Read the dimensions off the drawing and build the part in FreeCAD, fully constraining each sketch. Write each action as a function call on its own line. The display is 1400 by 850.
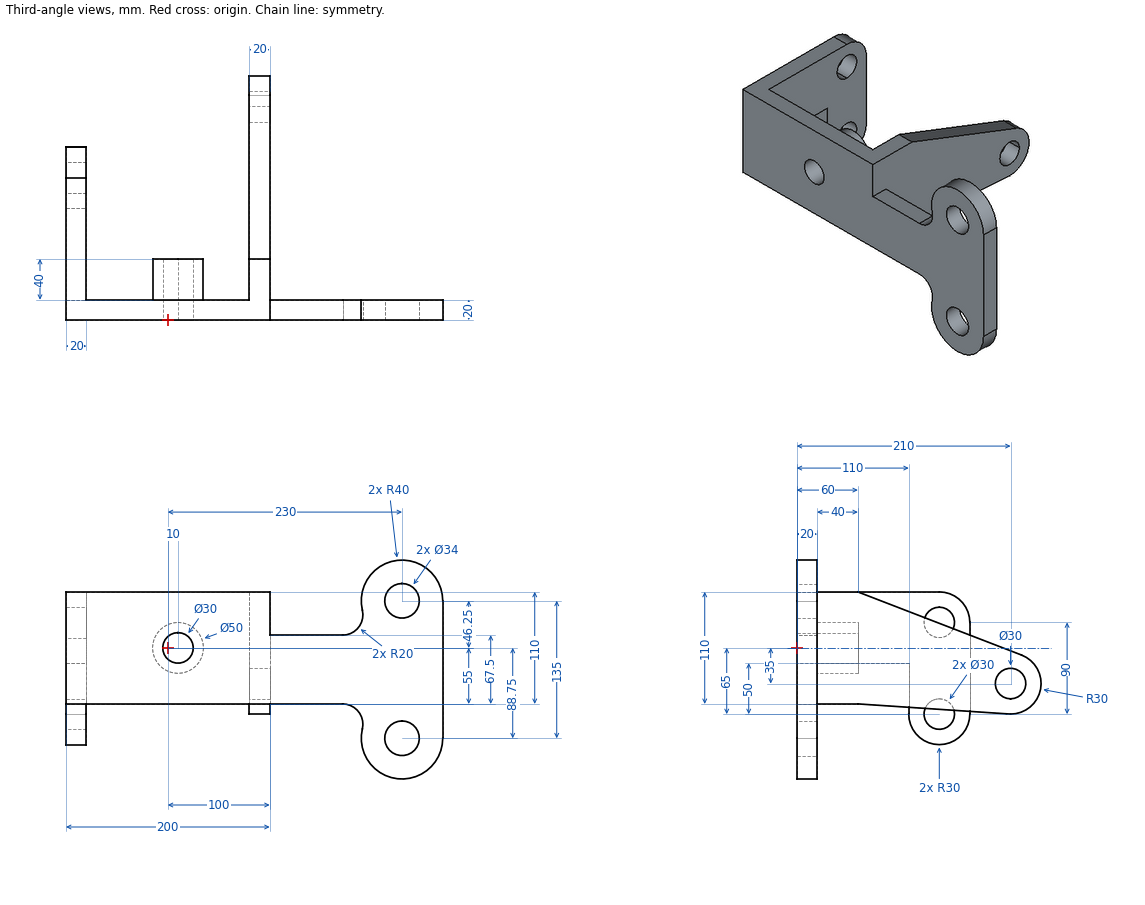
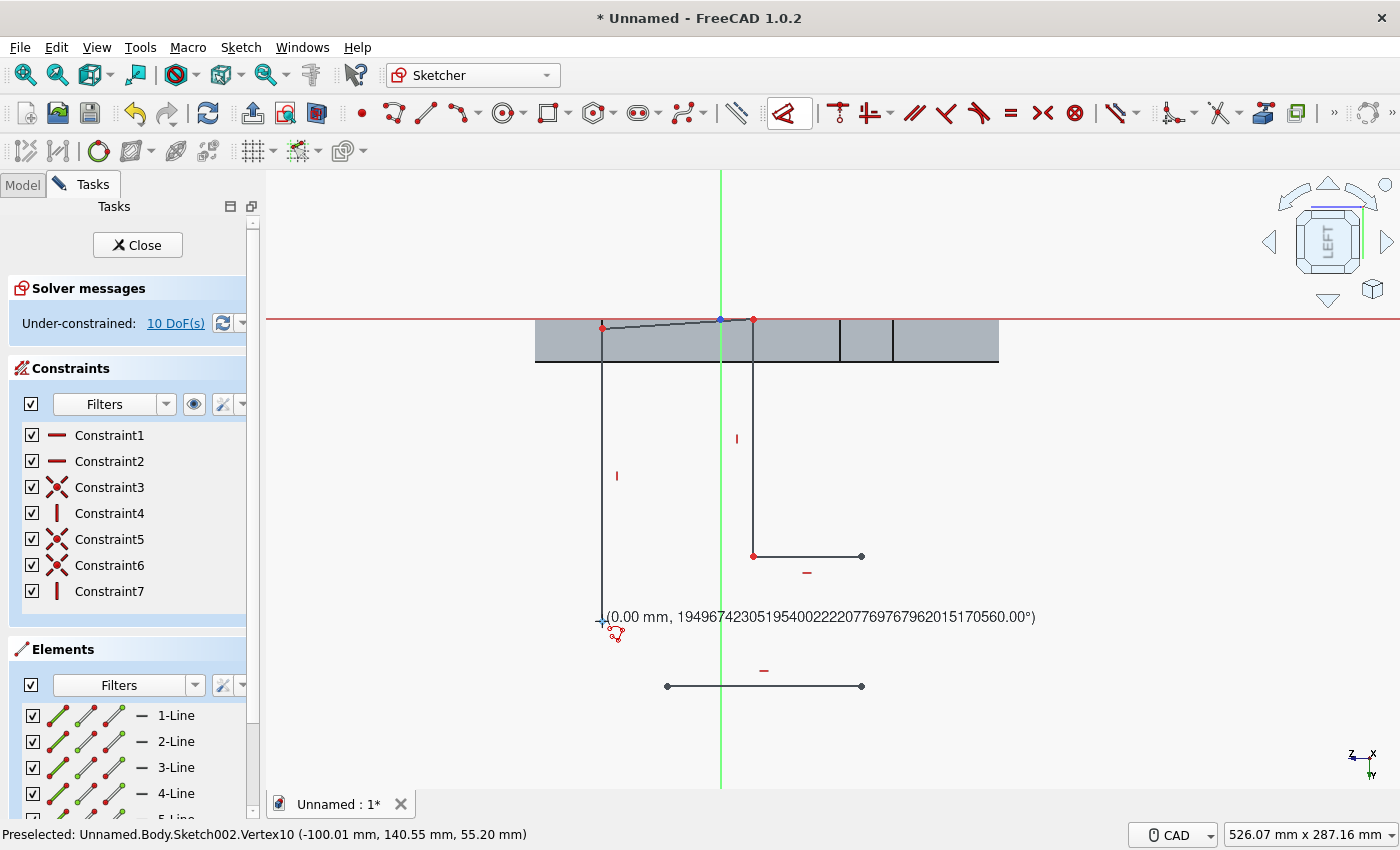
click(458, 114)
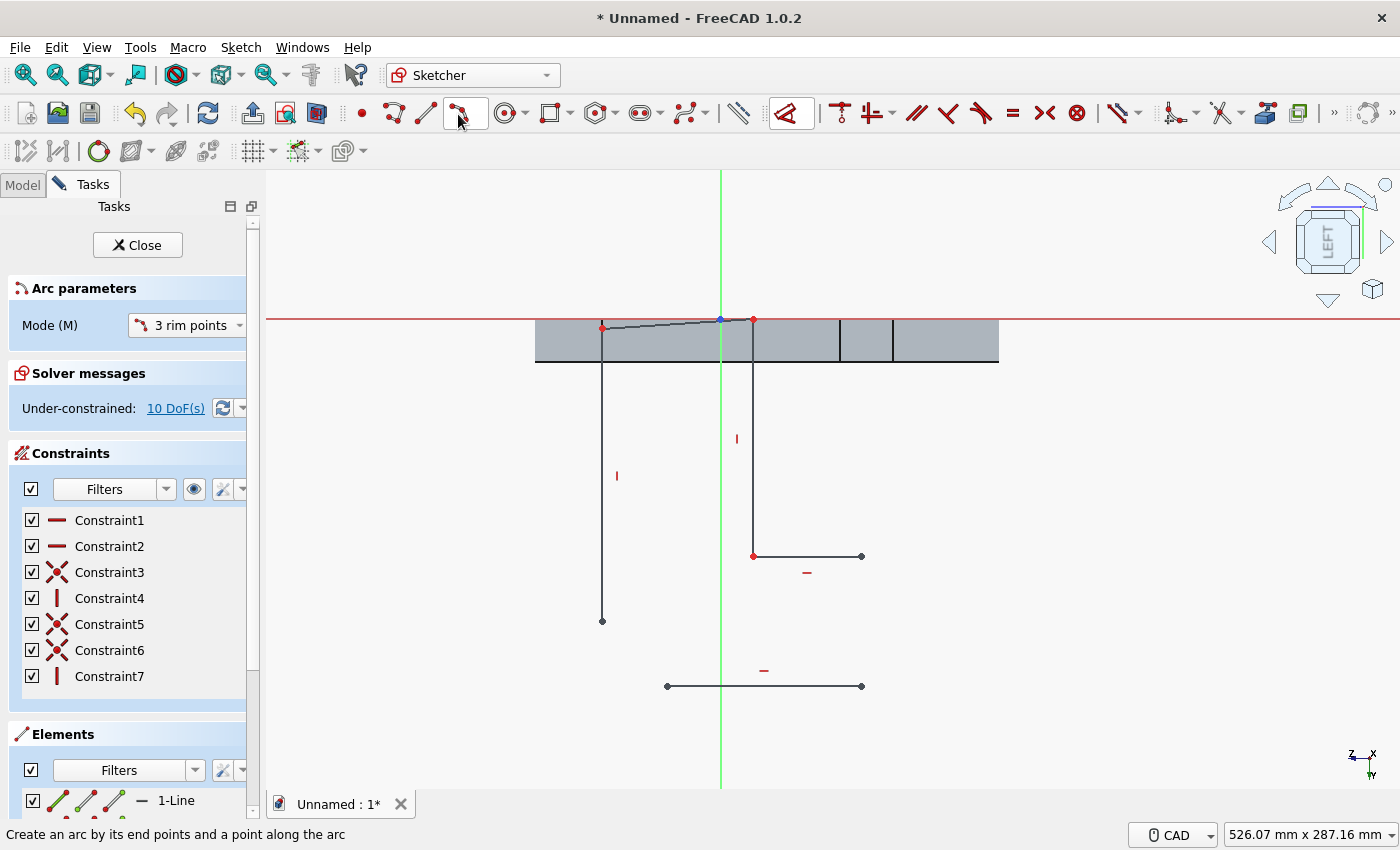
click(861, 686)
click(861, 557)
click(926, 621)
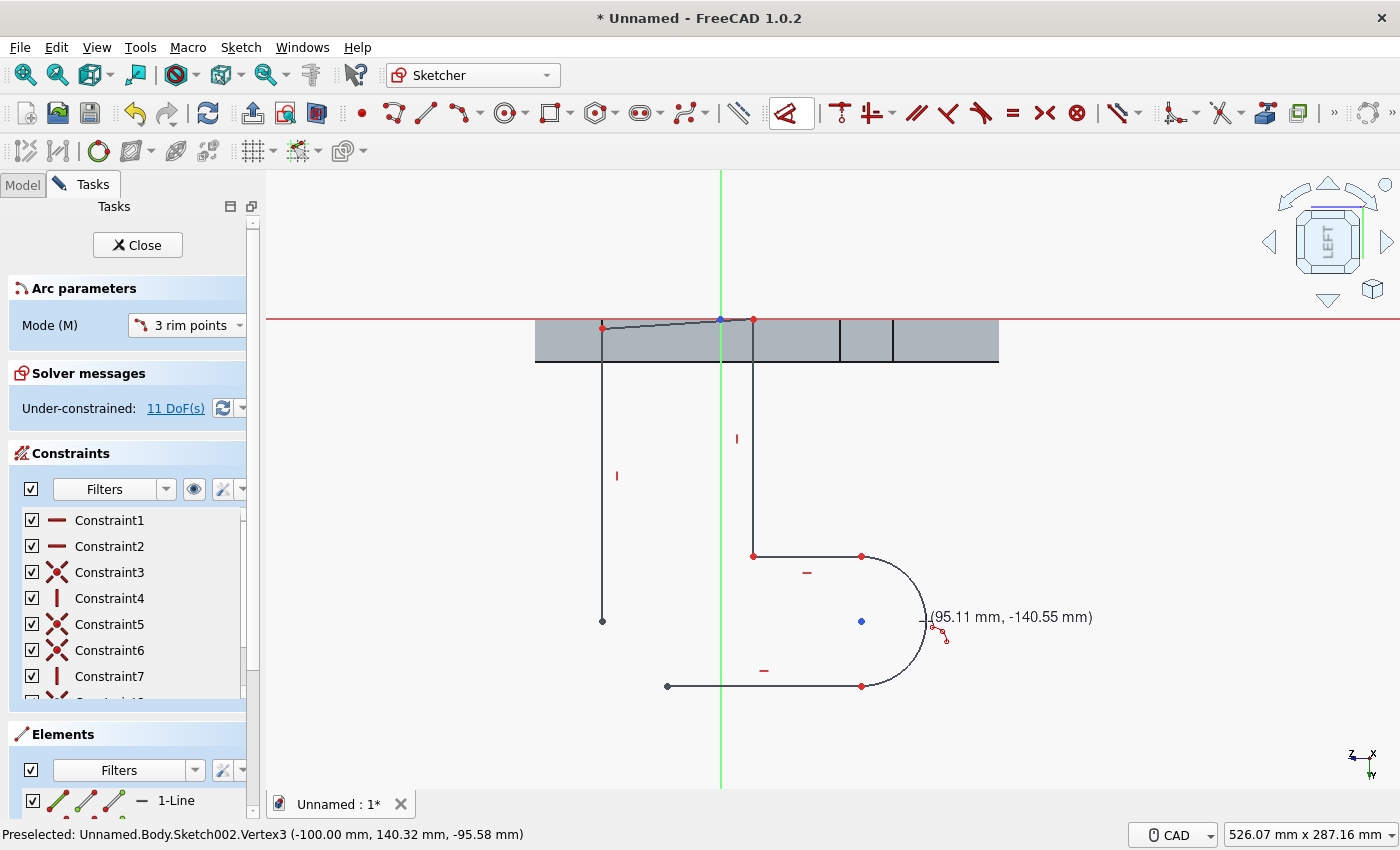
click(602, 622)
click(667, 686)
click(621, 667)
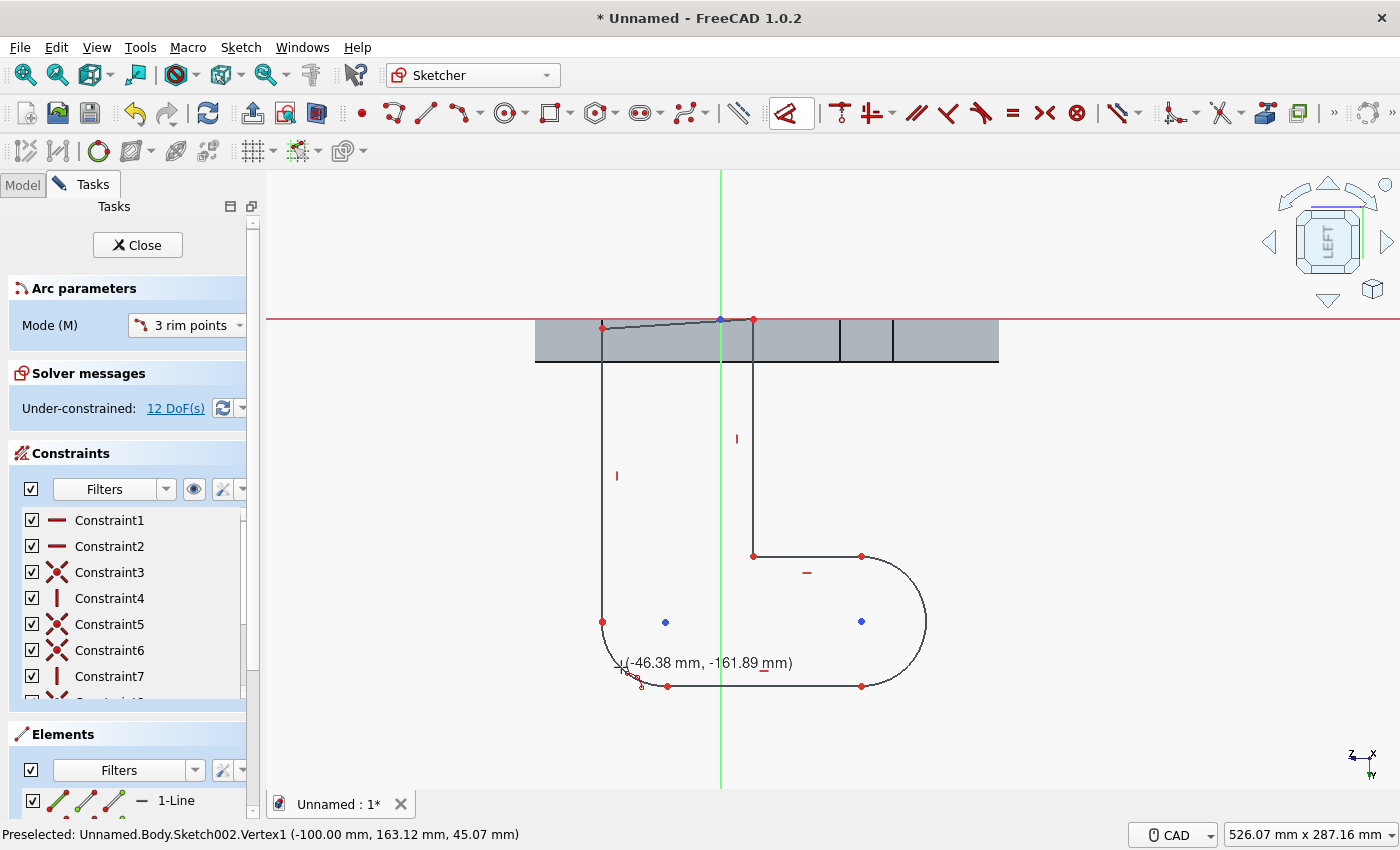
click(506, 114)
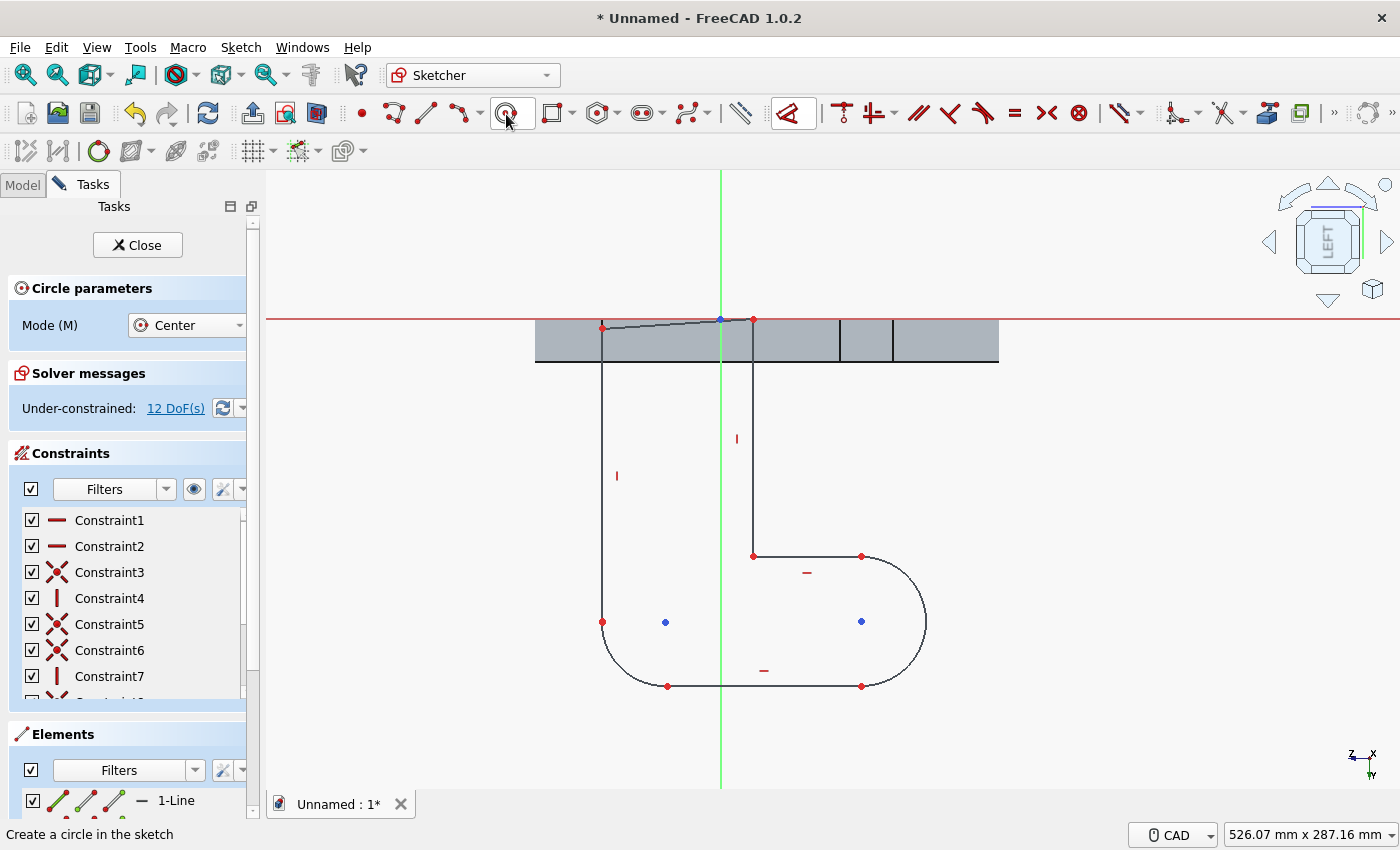
click(861, 621)
click(884, 598)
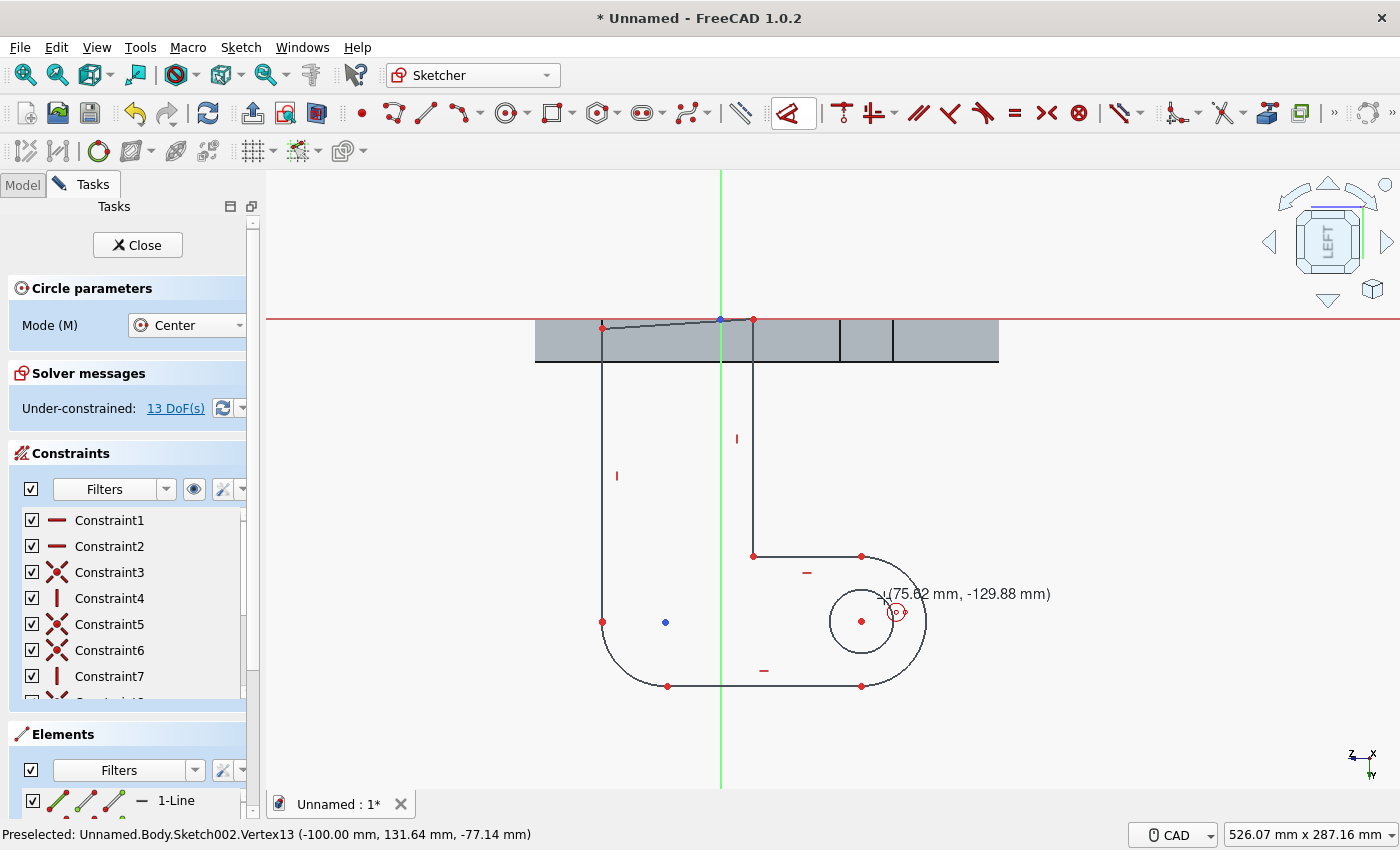
click(667, 621)
click(690, 598)
key(Escape)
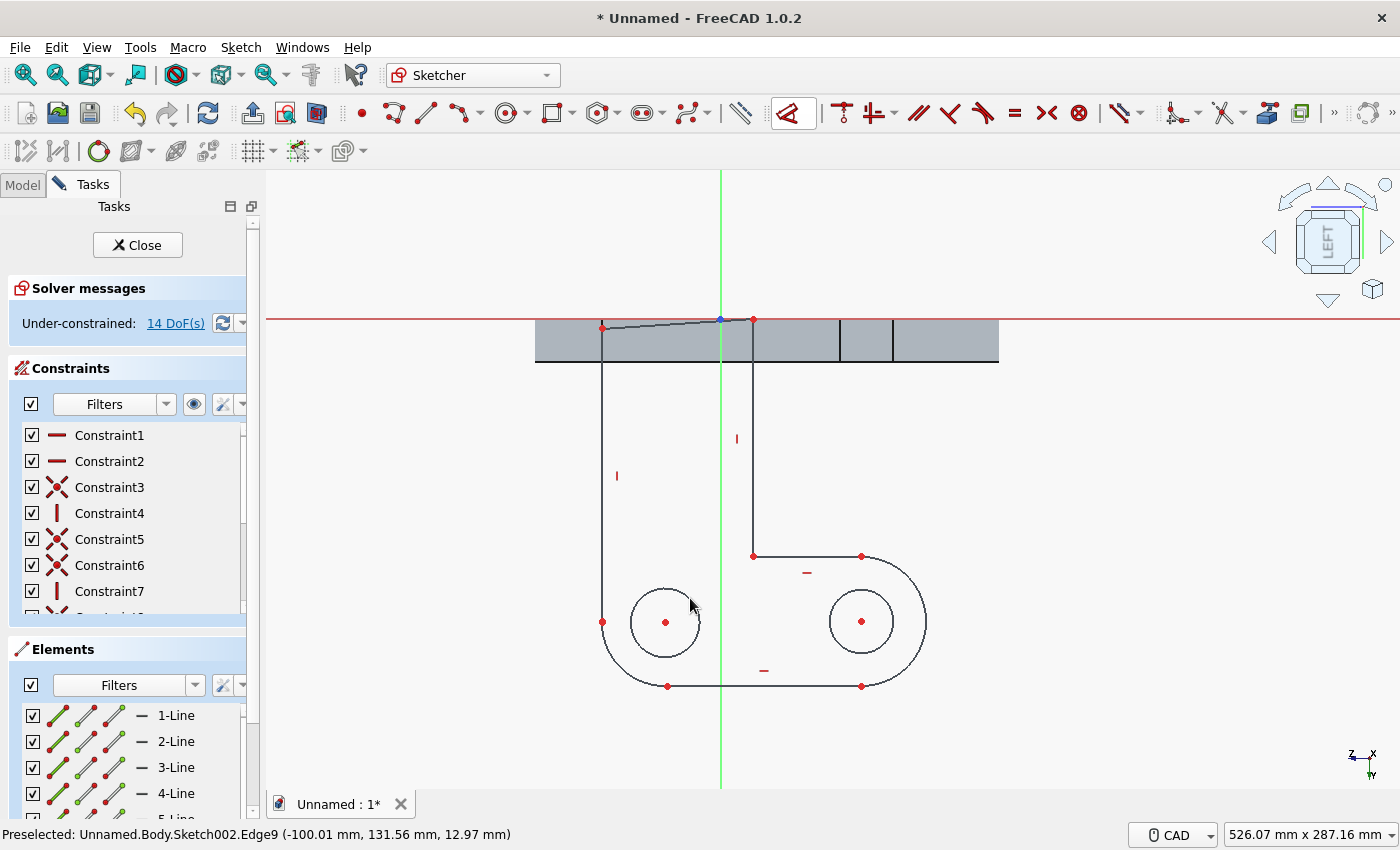
click(803, 686)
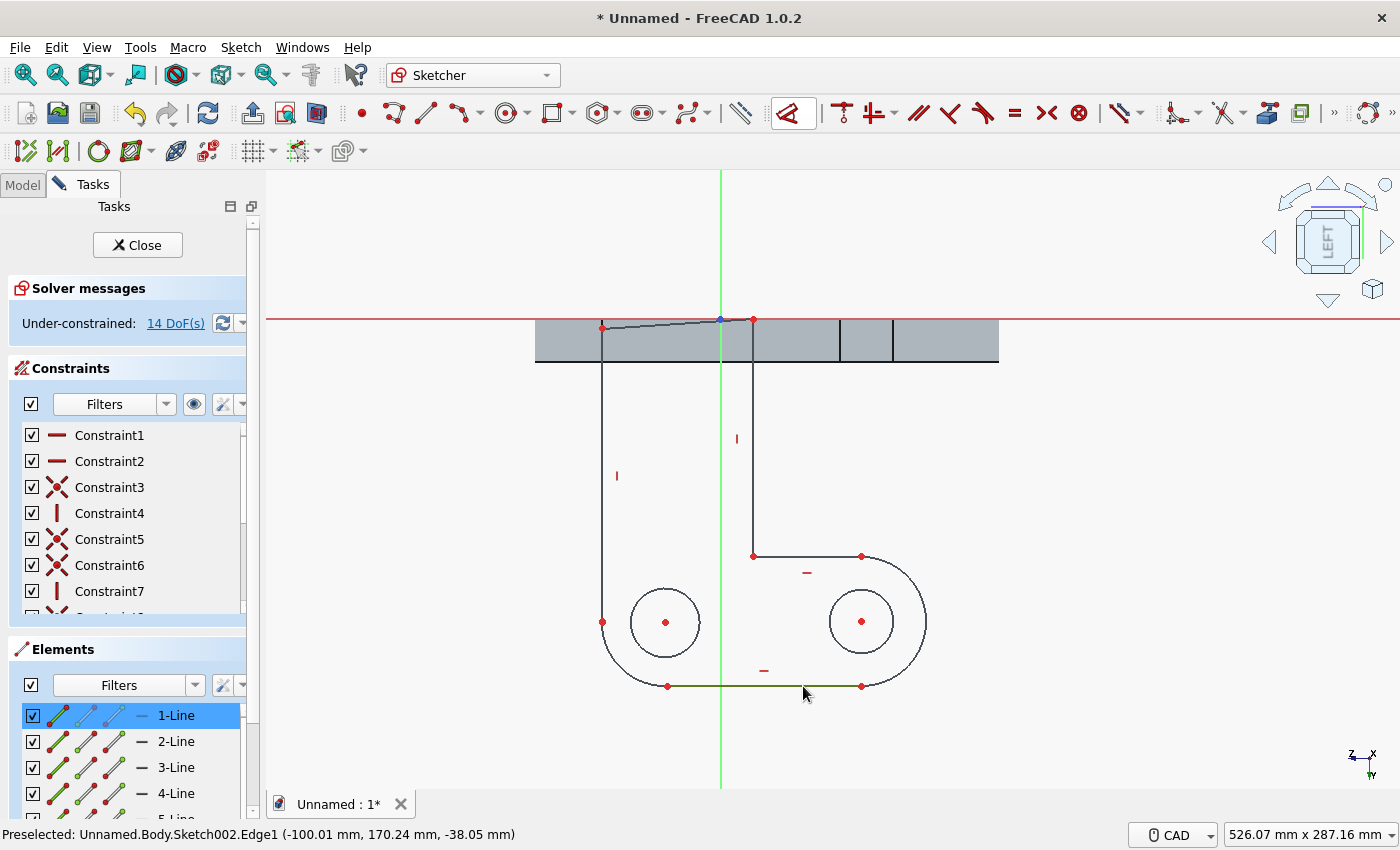
click(914, 660)